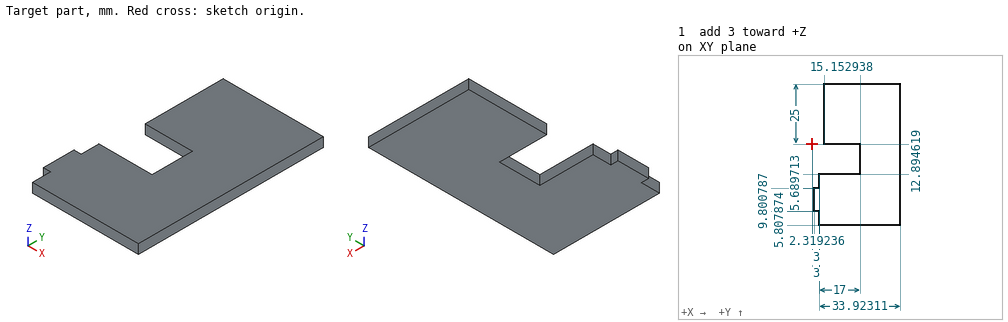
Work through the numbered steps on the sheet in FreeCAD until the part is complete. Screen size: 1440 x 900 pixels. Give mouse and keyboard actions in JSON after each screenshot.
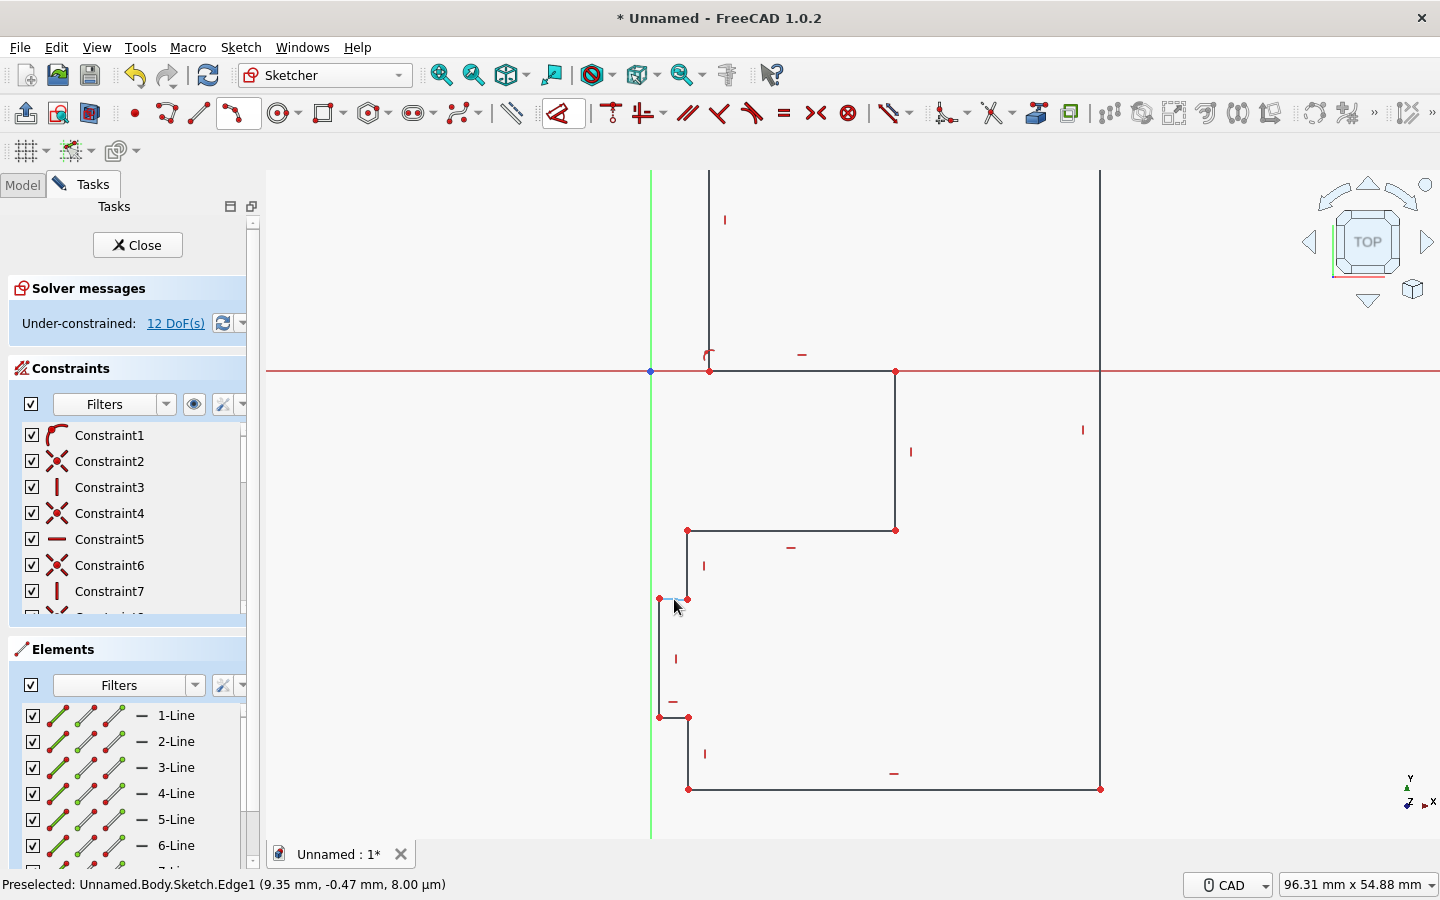
{"action": "left_click", "coordinate": [673, 599]}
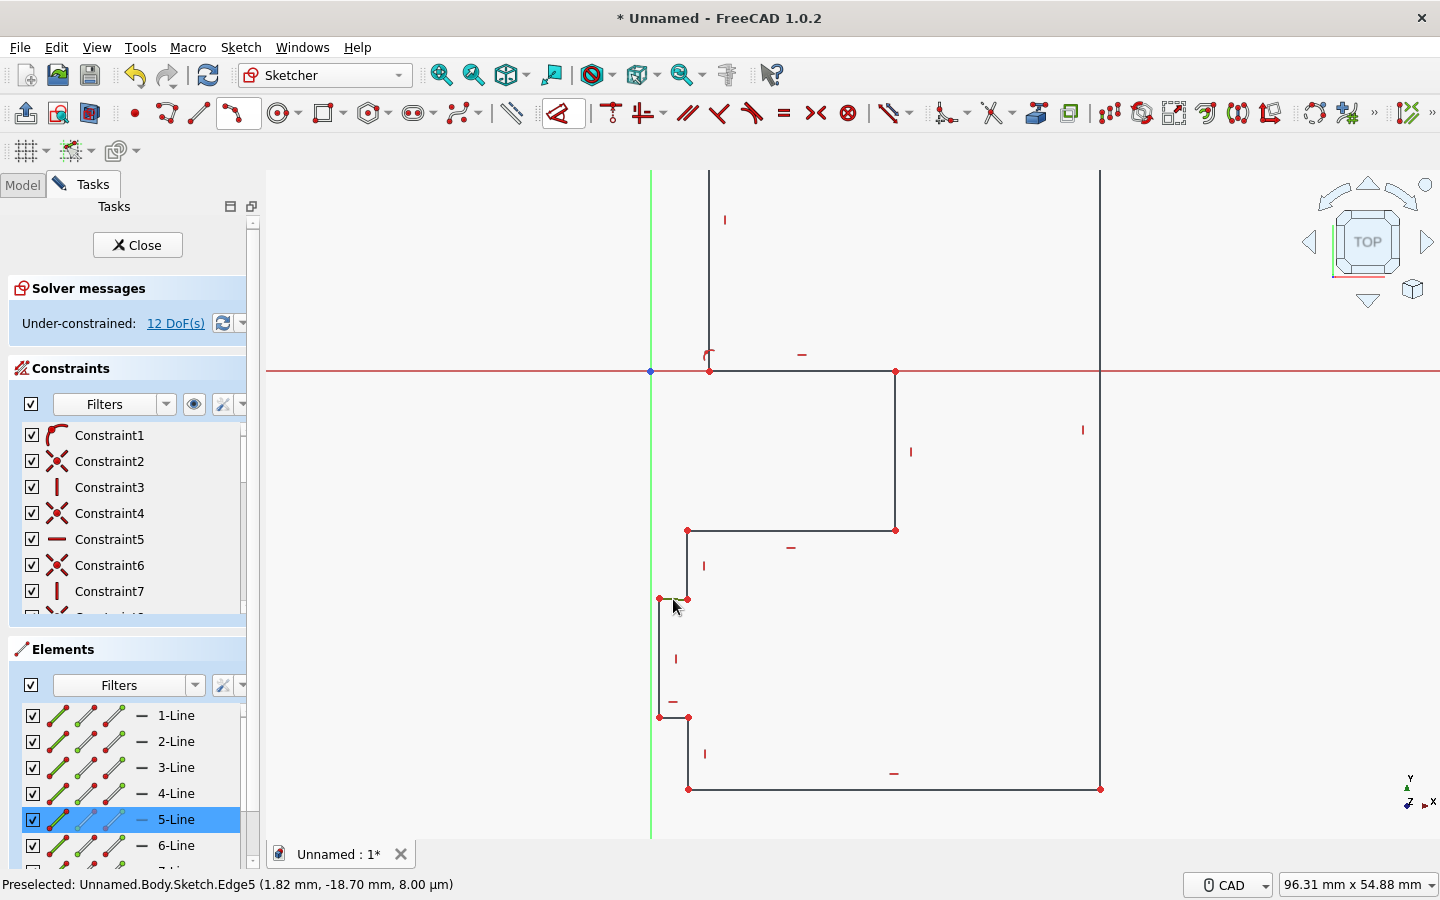
{"action": "key", "text": "h"}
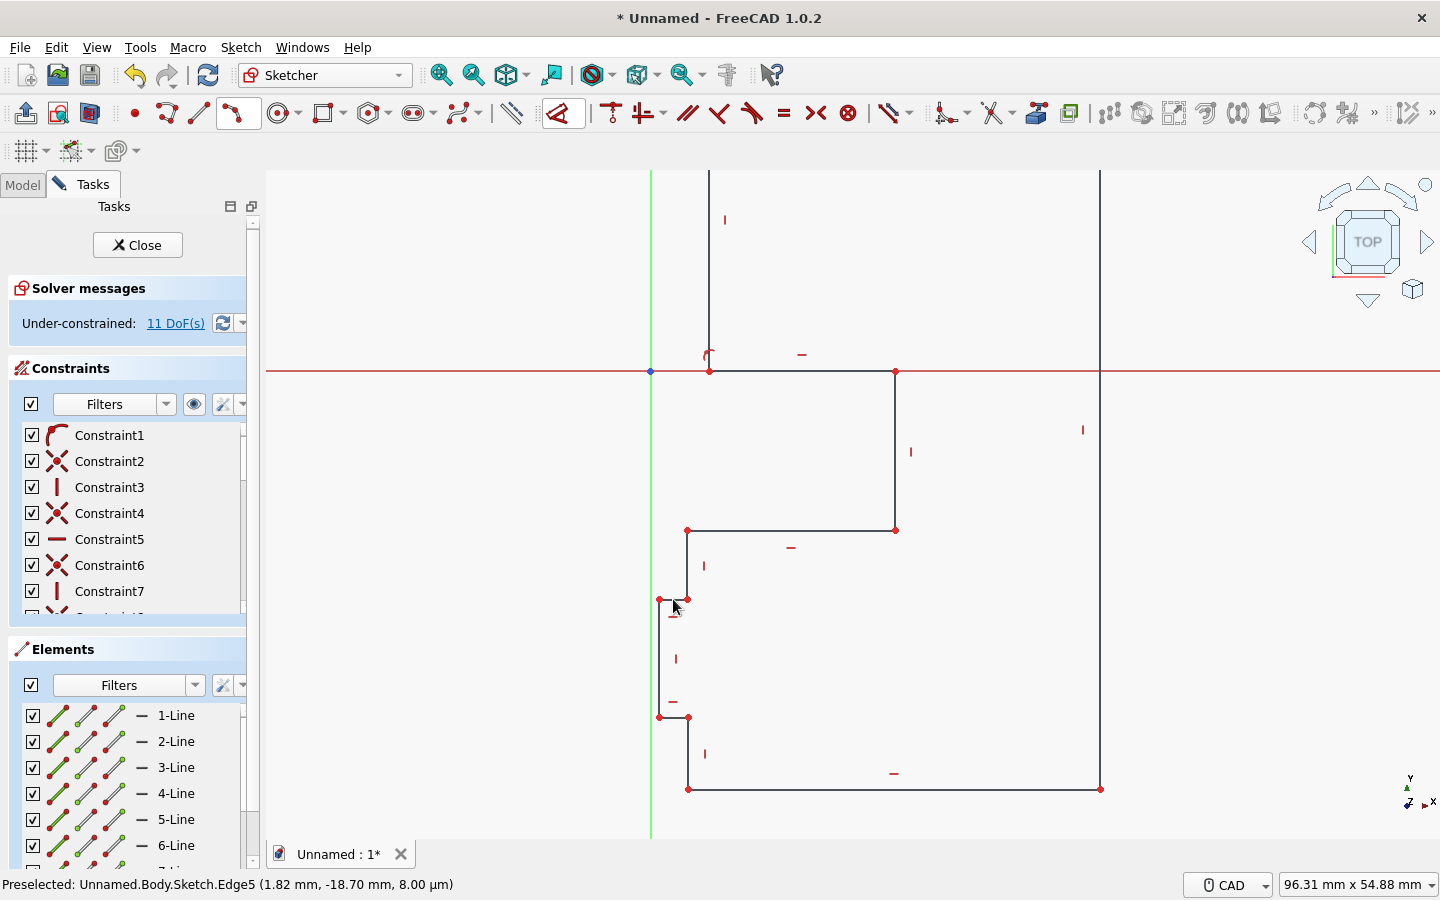
{"action": "left_click", "coordinate": [558, 114]}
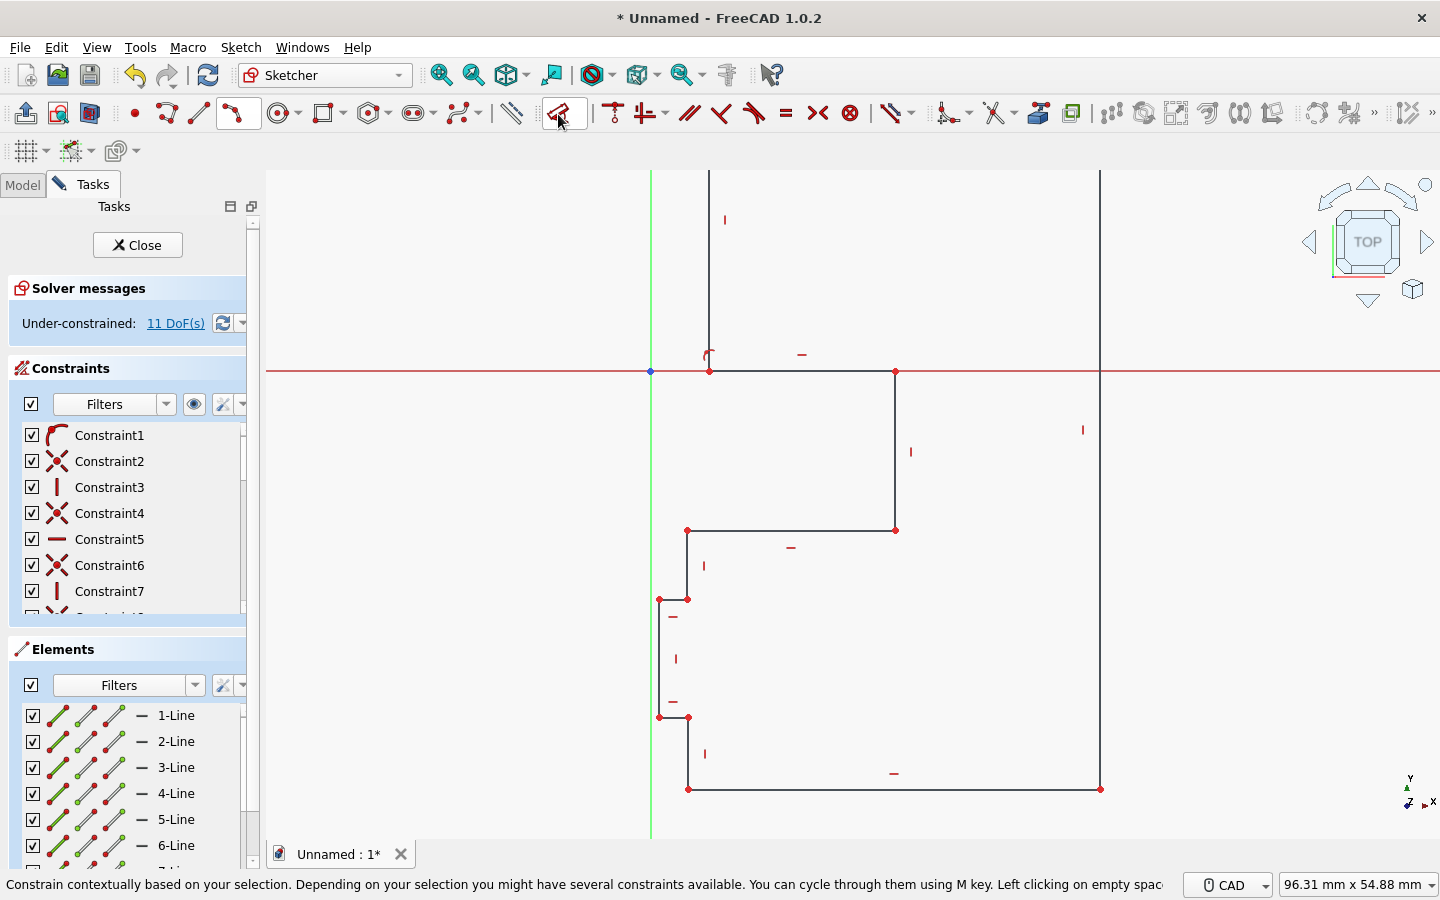
{"action": "left_click", "coordinate": [833, 531]}
{"action": "left_click", "coordinate": [791, 565]}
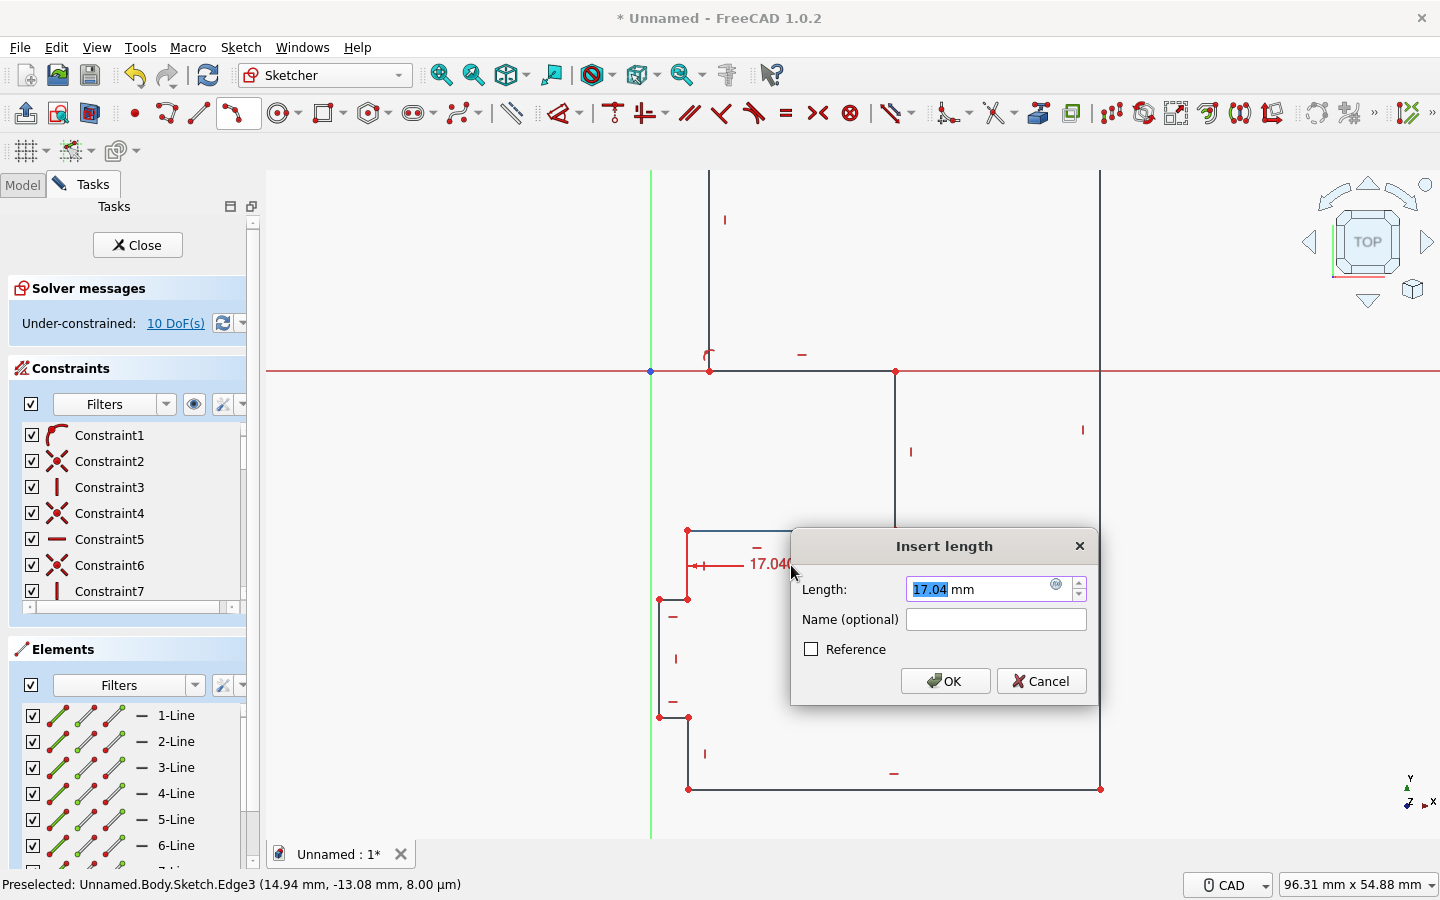
{"action": "type", "text": "17"}
{"action": "key", "text": "Return"}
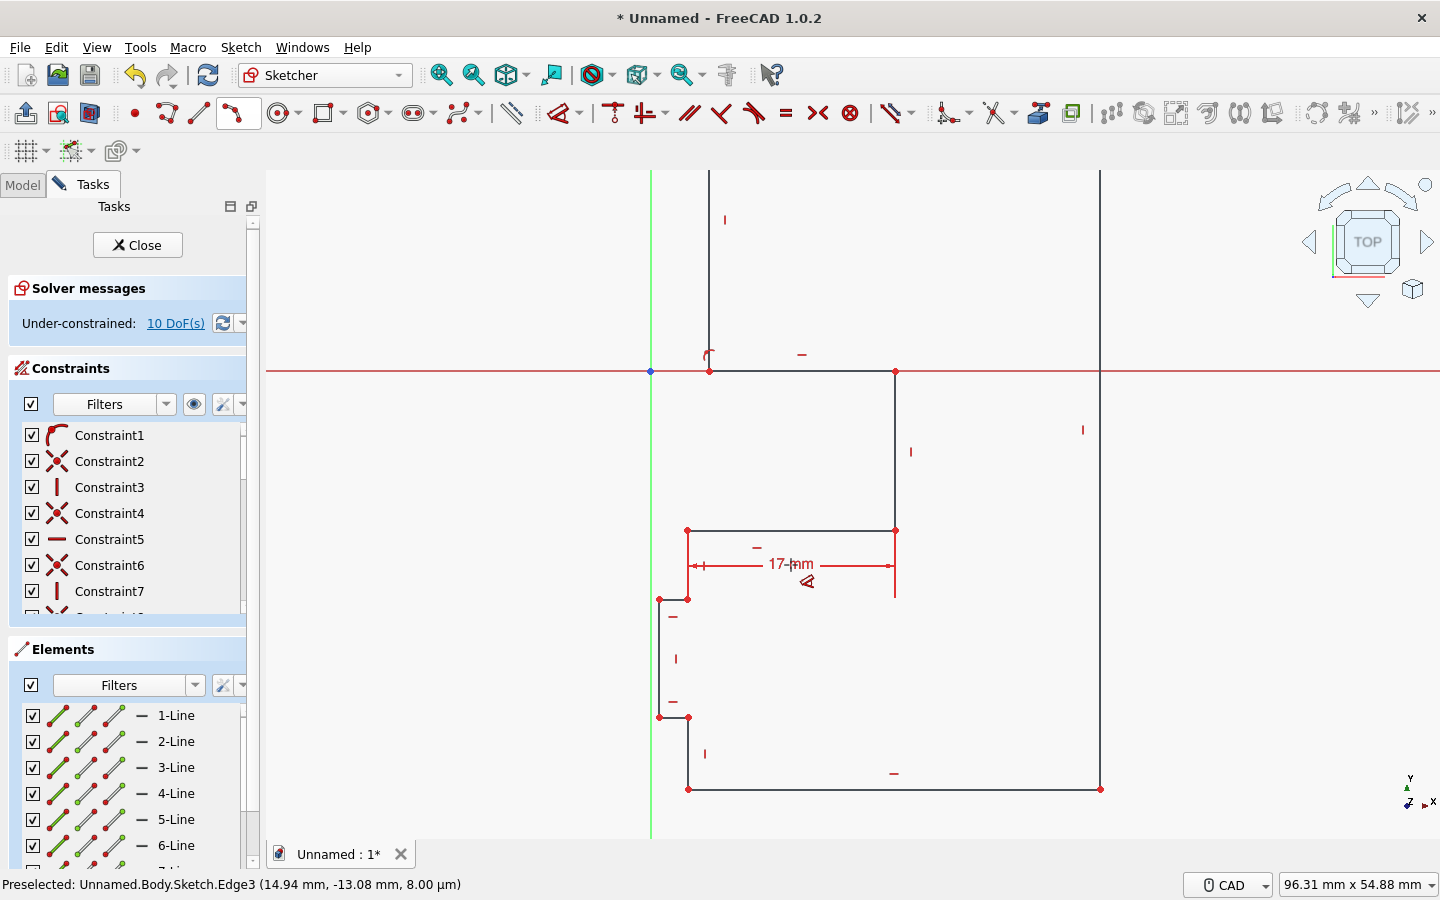
{"action": "left_click", "coordinate": [709, 280]}
{"action": "left_click", "coordinate": [675, 285]}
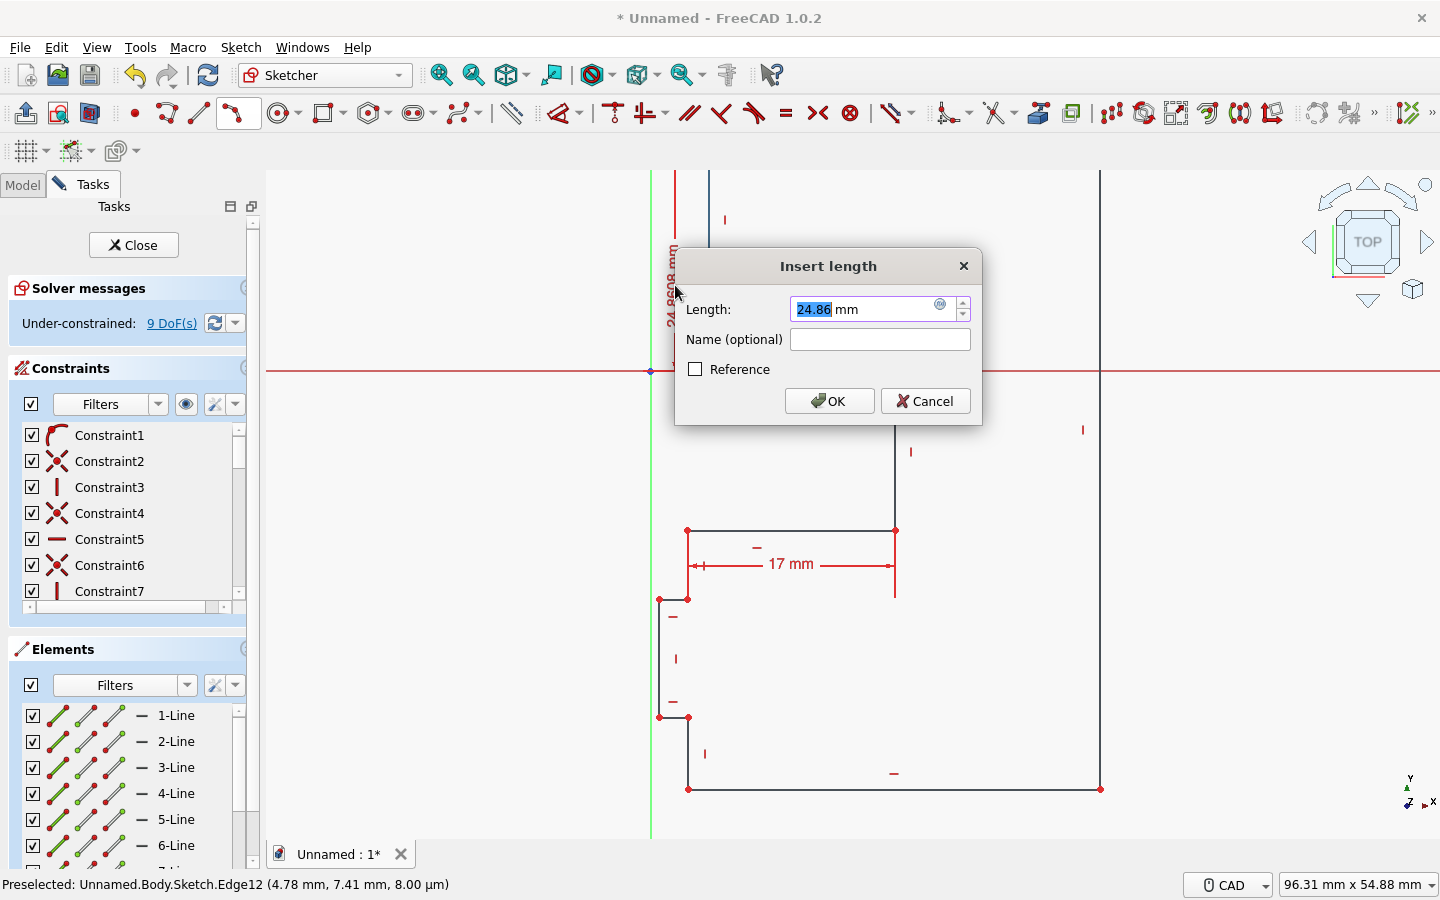
{"action": "type", "text": "25"}
{"action": "key", "text": "Return"}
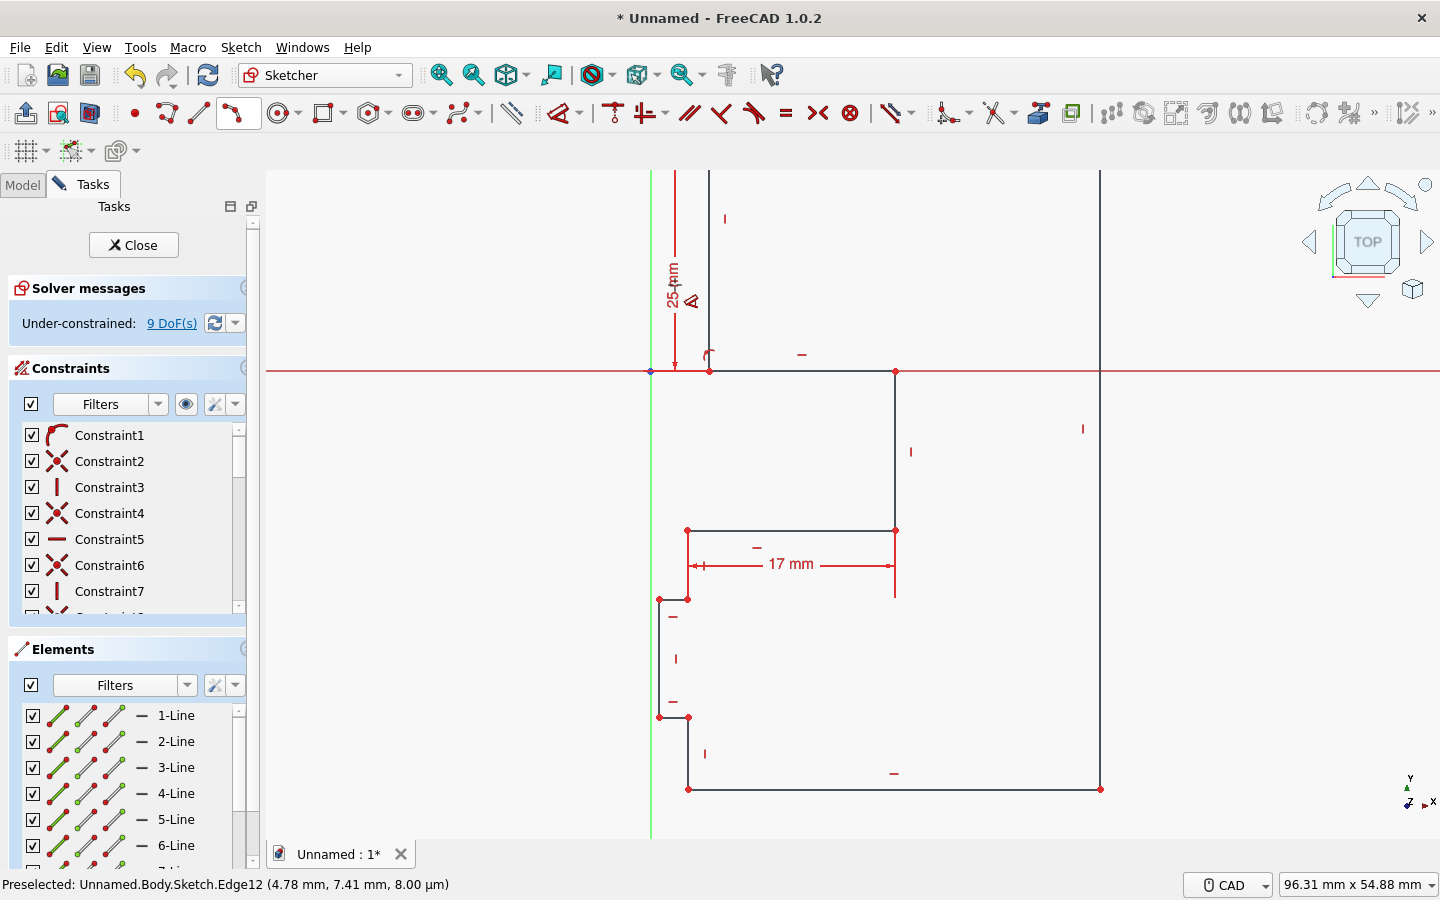
{"action": "left_click", "coordinate": [688, 531]}
{"action": "left_click", "coordinate": [669, 565]}